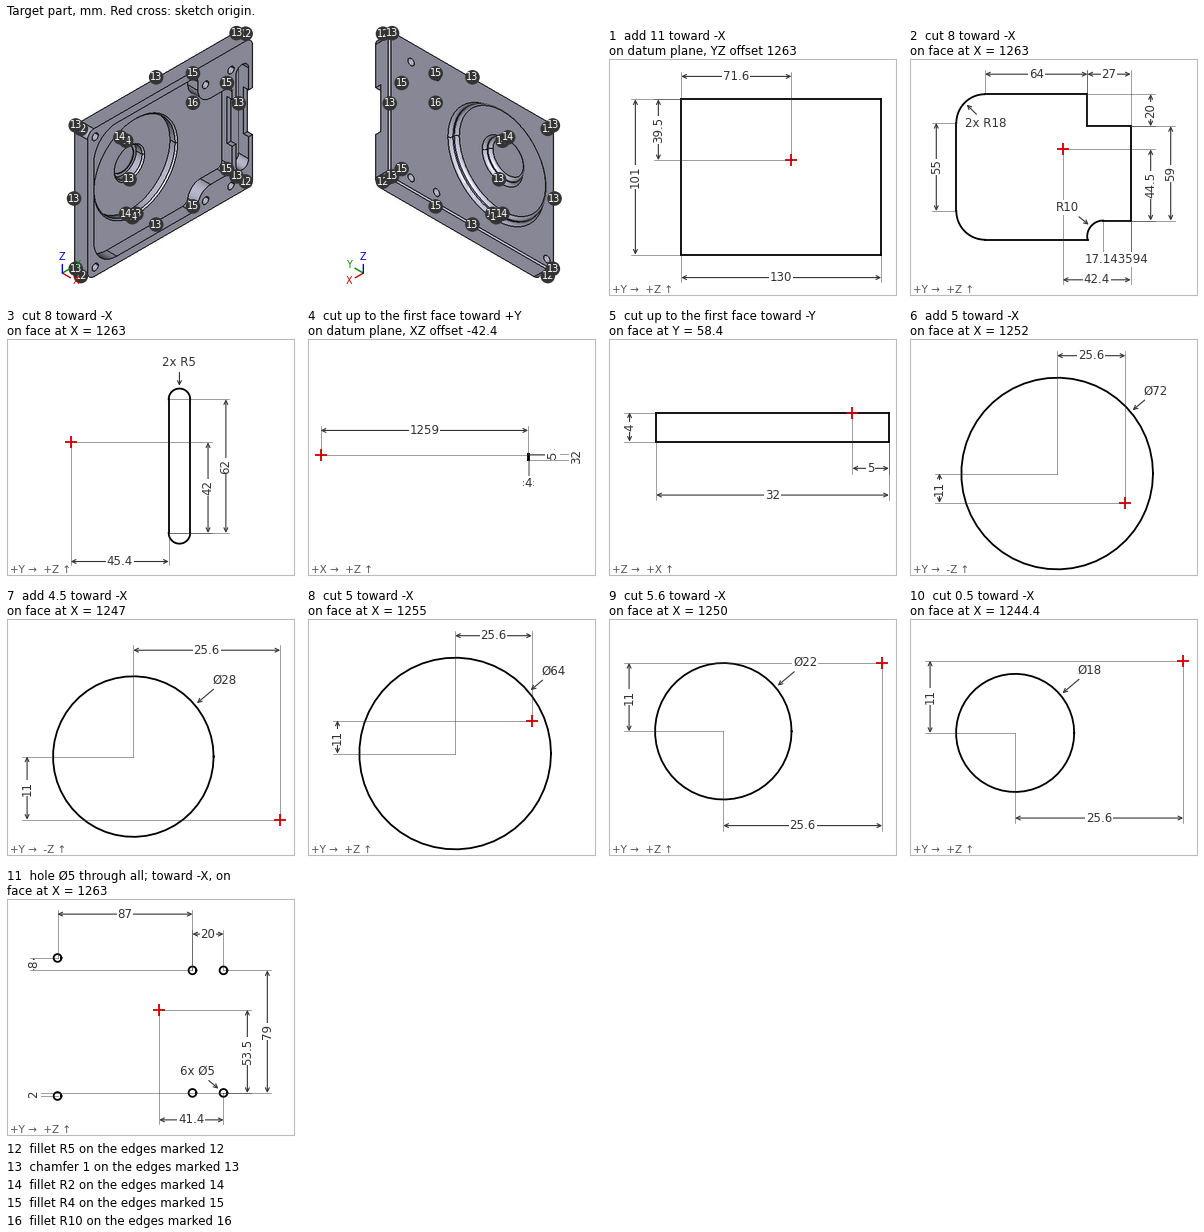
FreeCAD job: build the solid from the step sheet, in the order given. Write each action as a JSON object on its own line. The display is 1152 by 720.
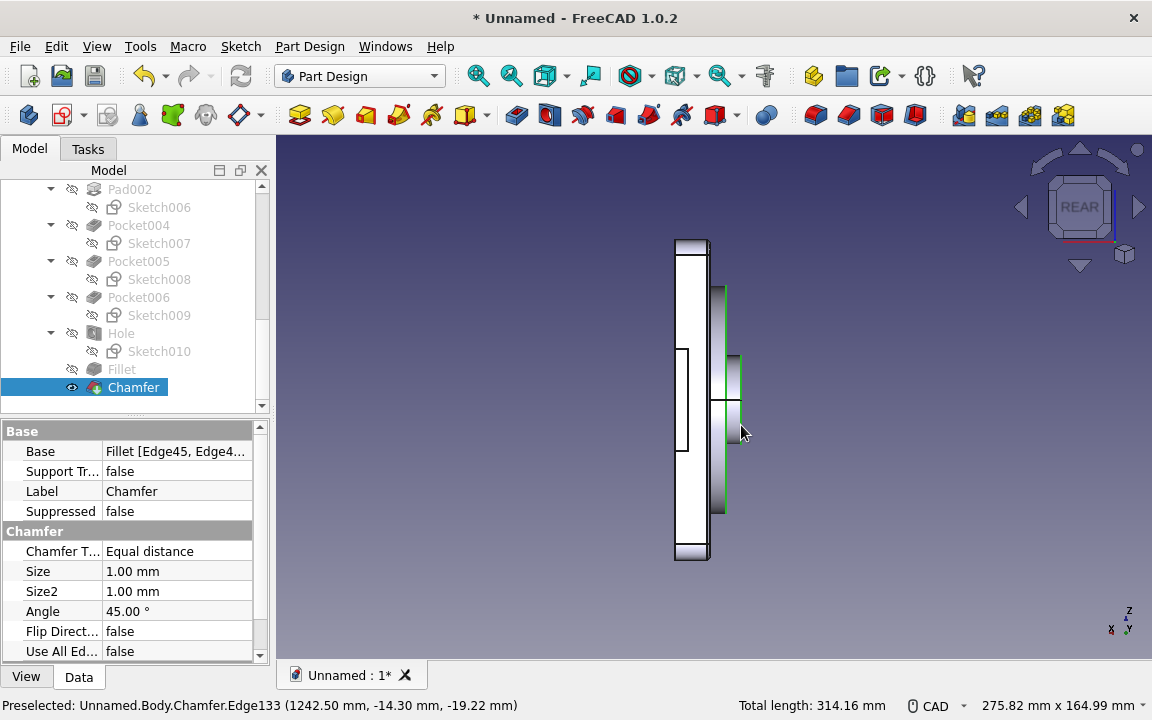
{"action": "key", "text": "6"}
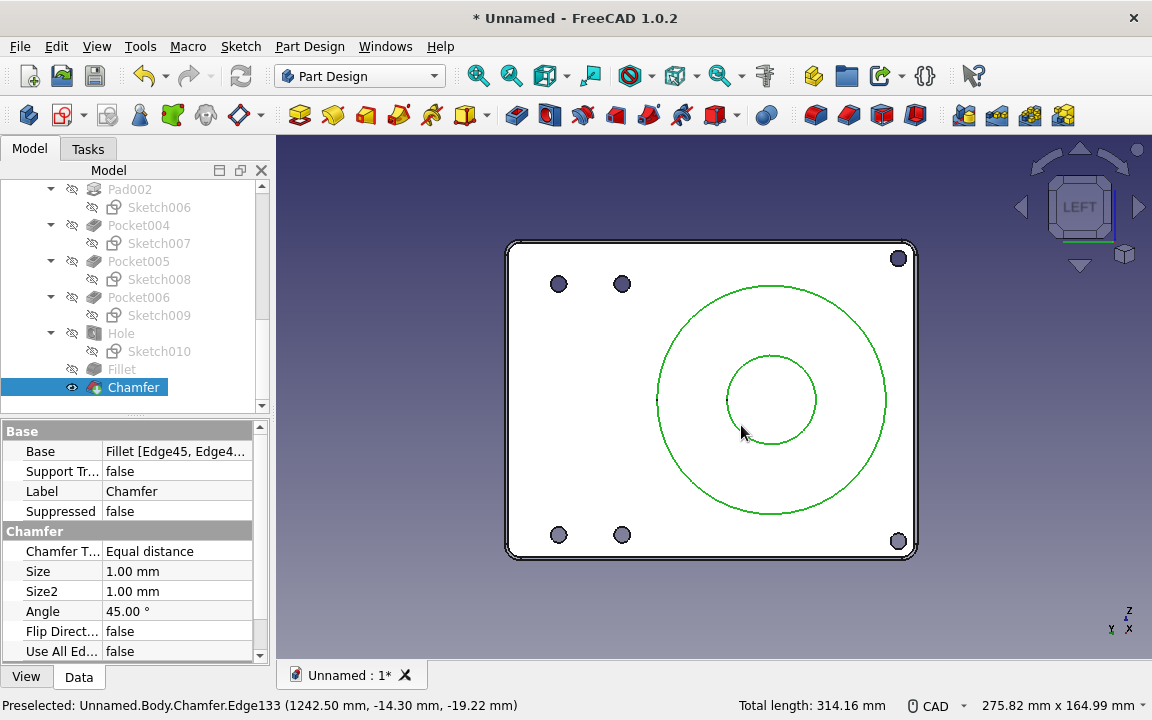
{"action": "key", "text": "v 3"}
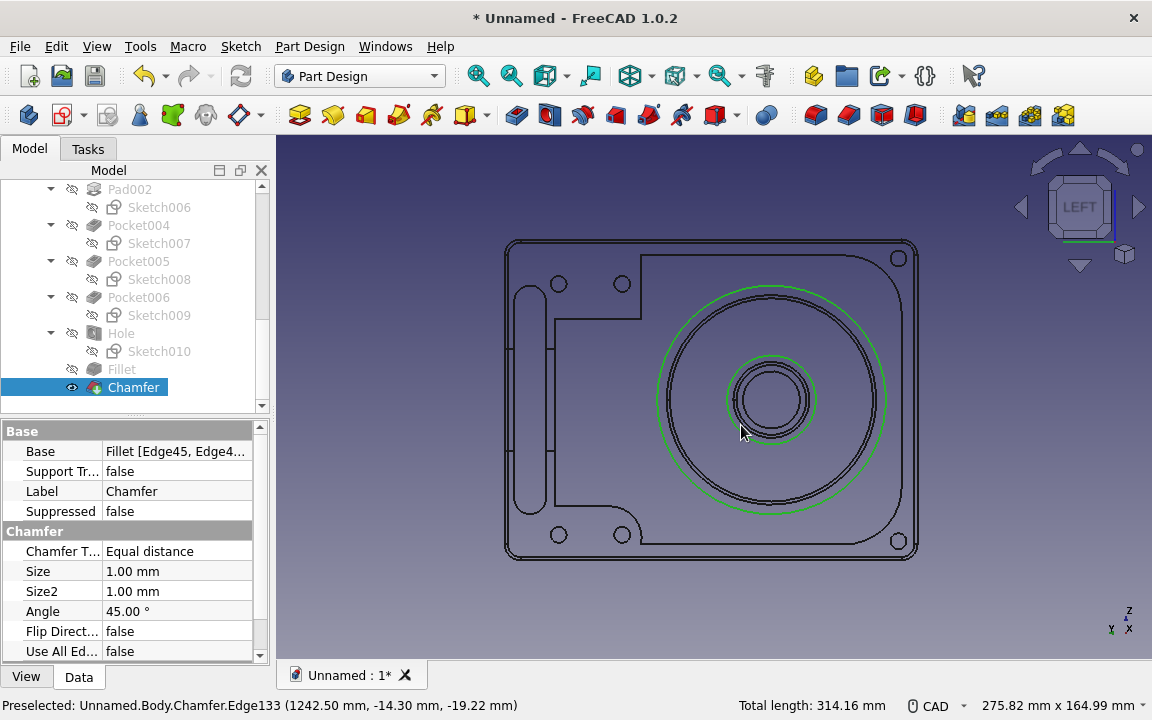
{"action": "key", "text": "0"}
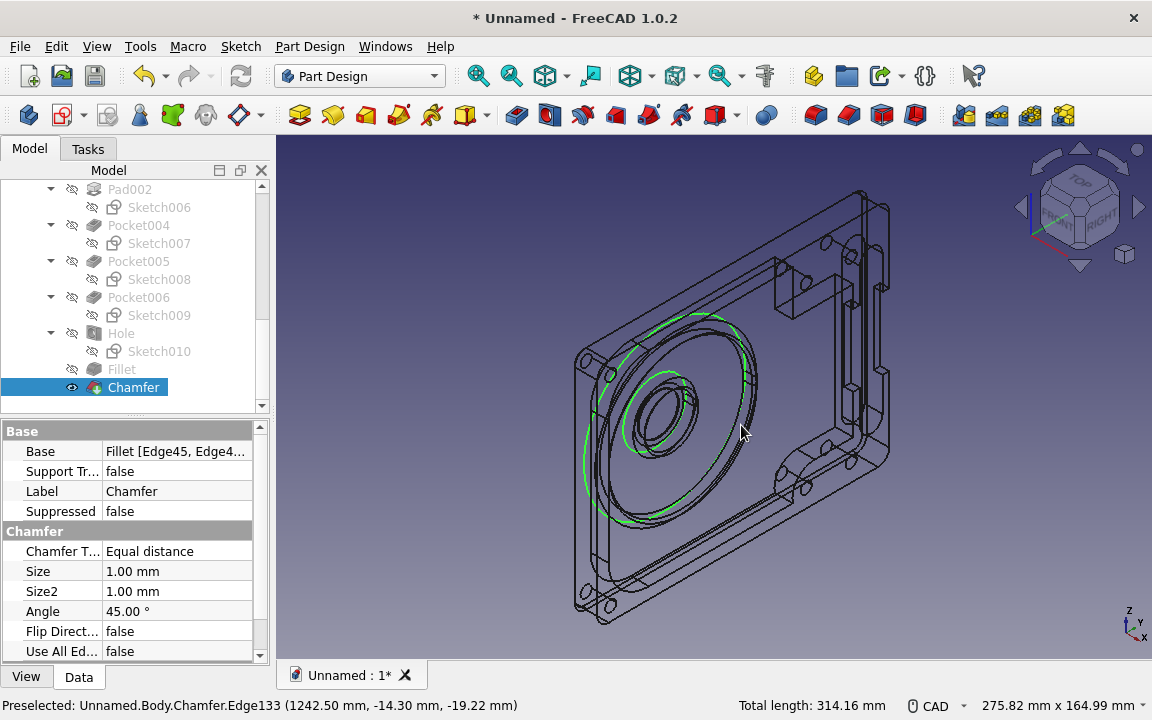
{"action": "left_click", "coordinate": [735, 325], "text": "ctrl"}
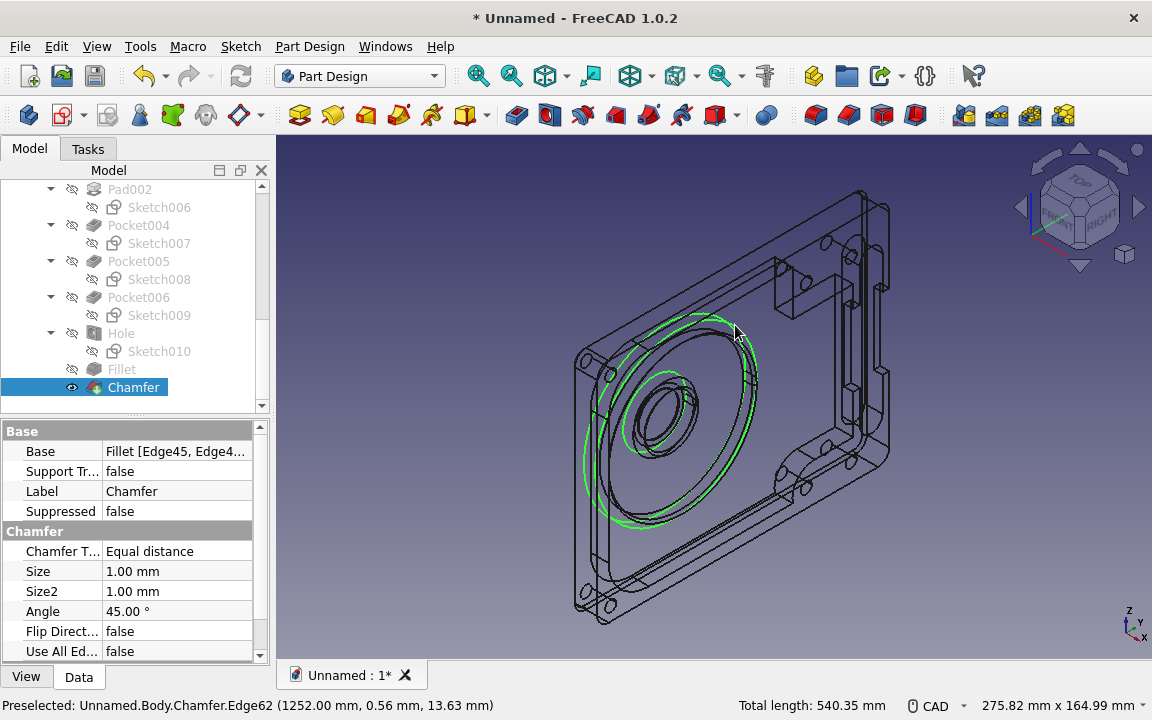
{"action": "left_click", "coordinate": [633, 435], "text": "ctrl"}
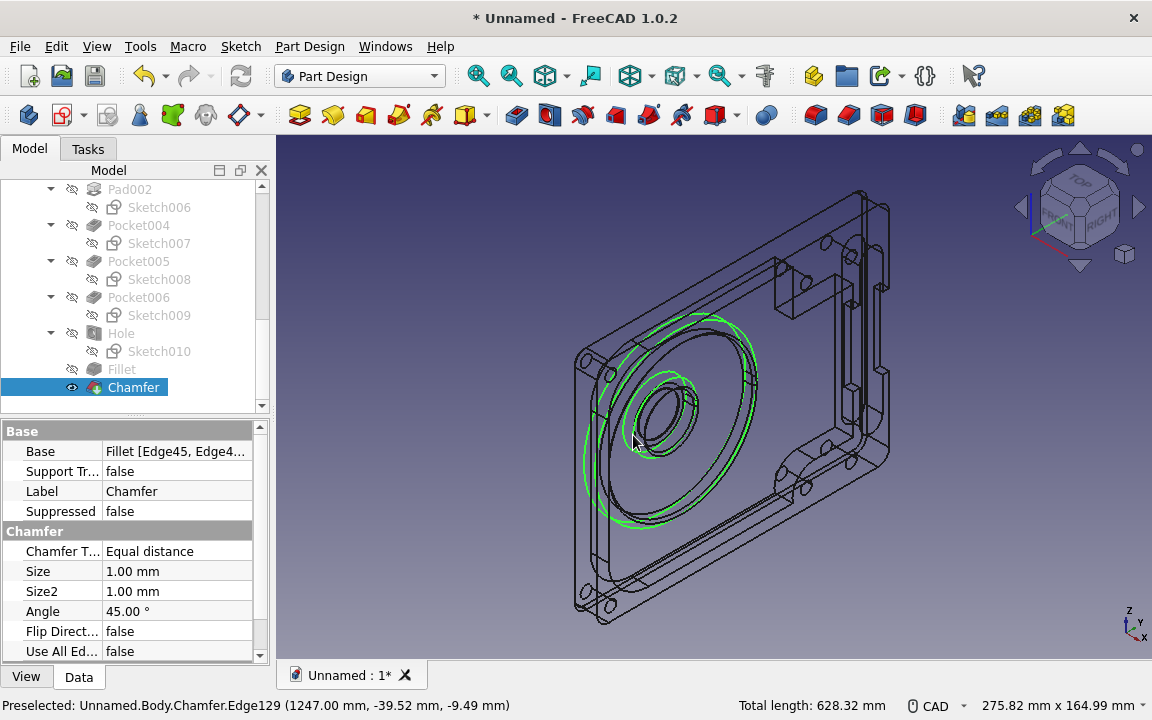
{"action": "key", "text": "v 1"}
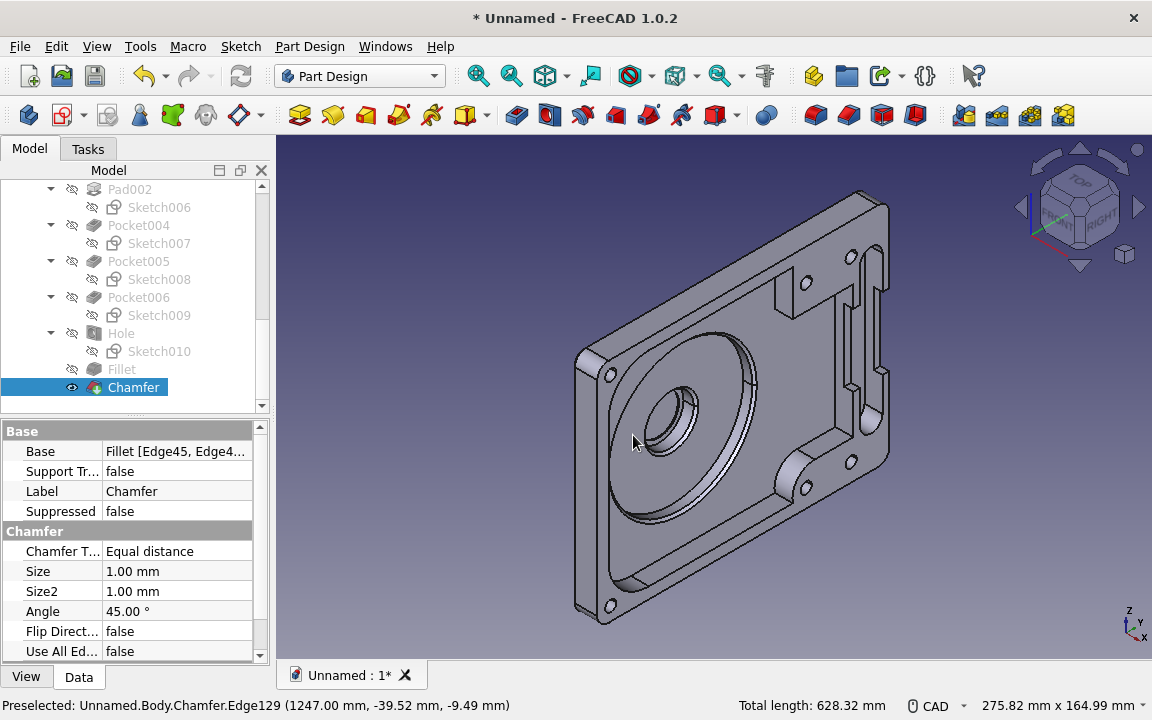
{"action": "left_click", "coordinate": [816, 116]}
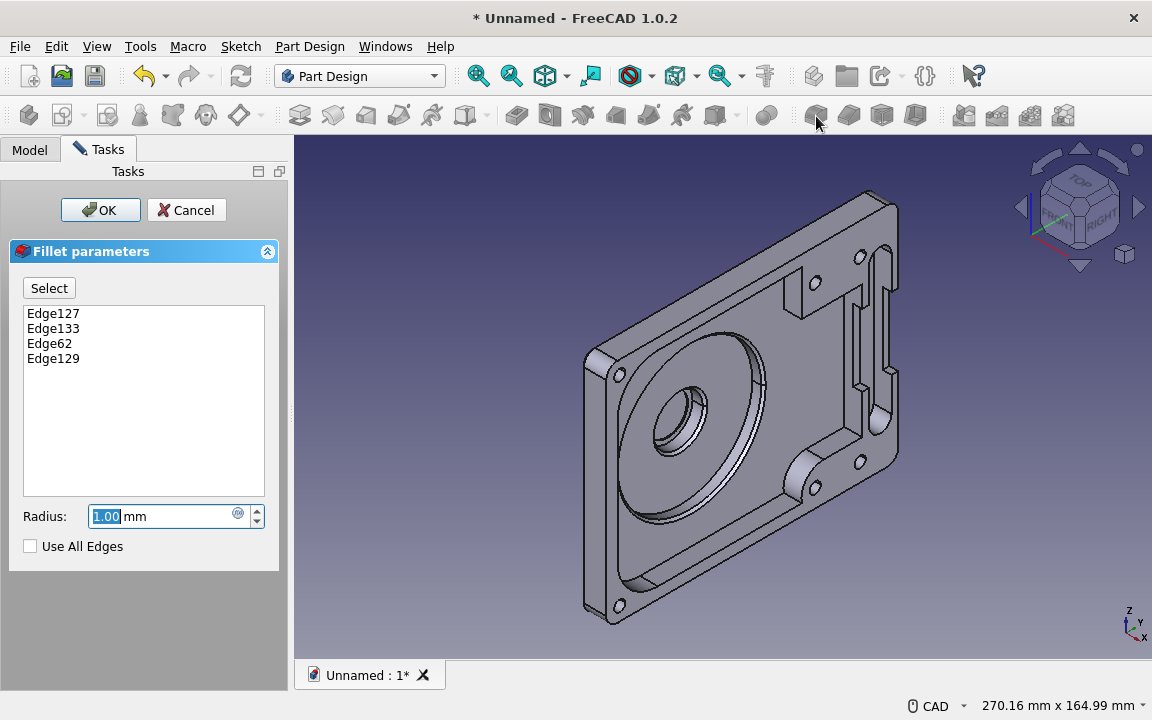
{"action": "type", "text": "2"}
{"action": "key", "text": "Tab"}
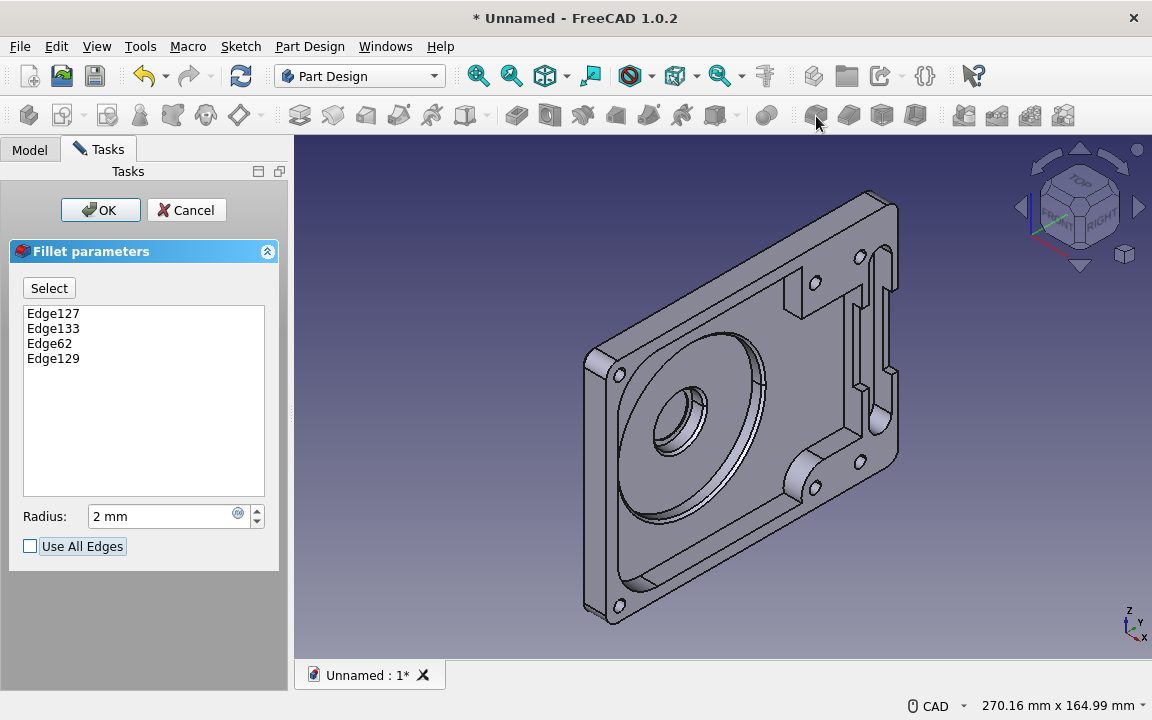
{"action": "left_click", "coordinate": [101, 210]}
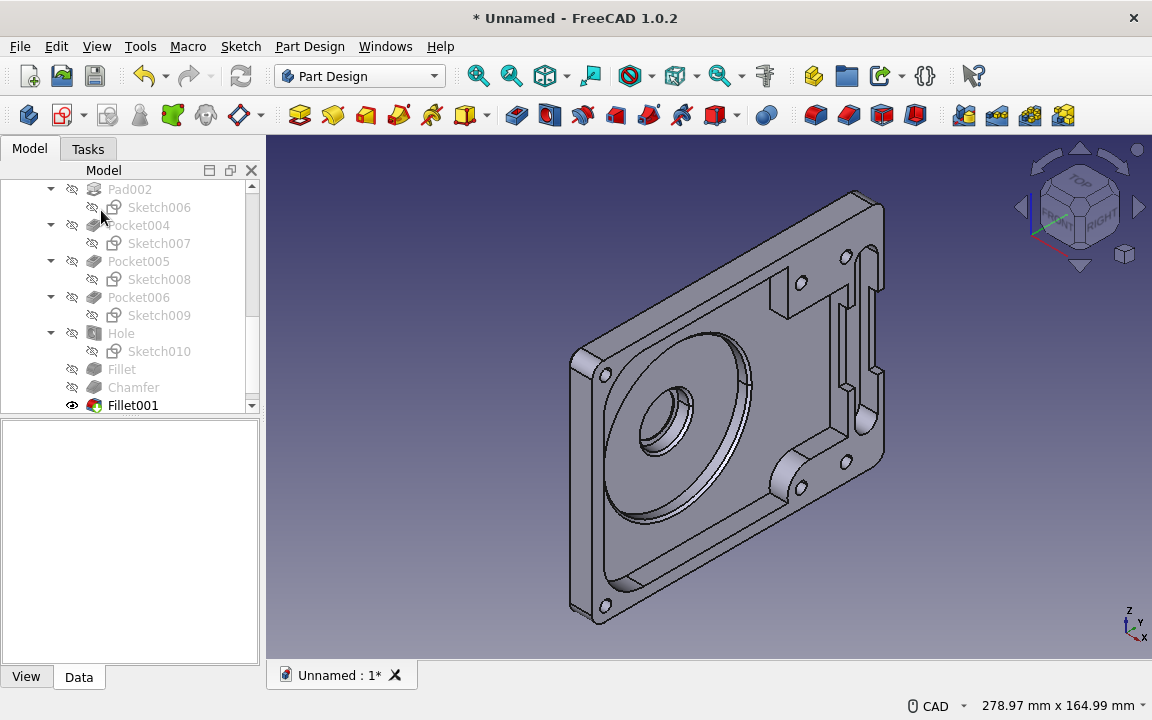
{"action": "key", "text": "2"}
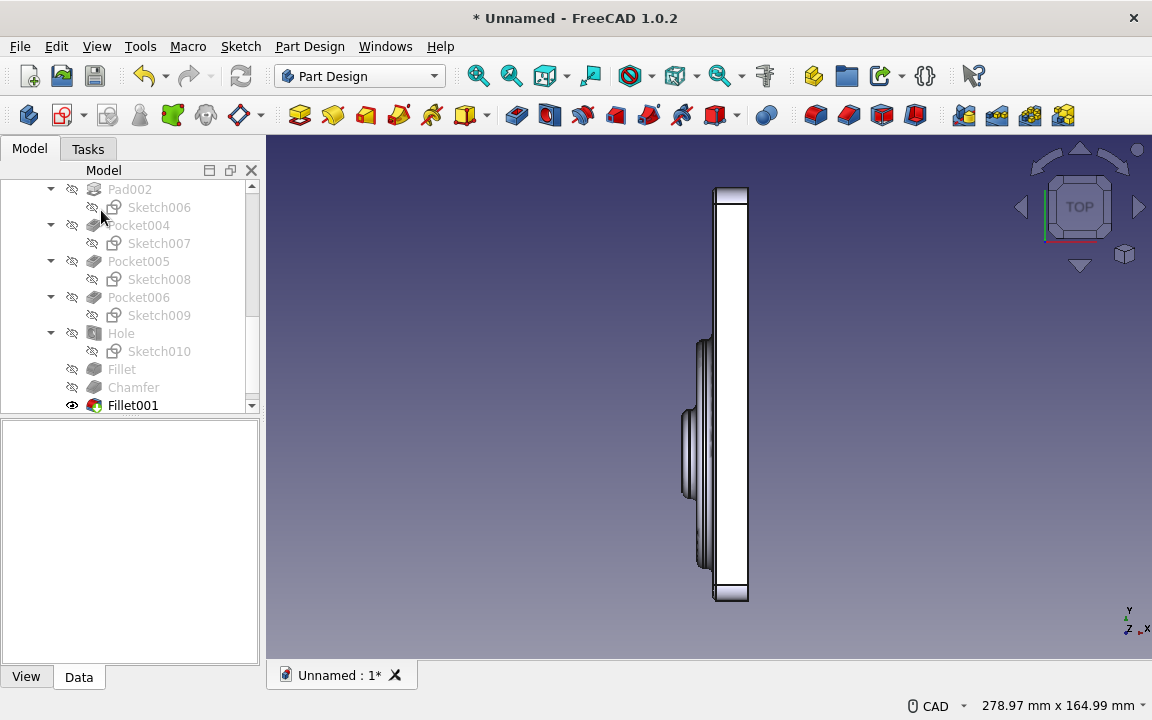
{"action": "key", "text": "0"}